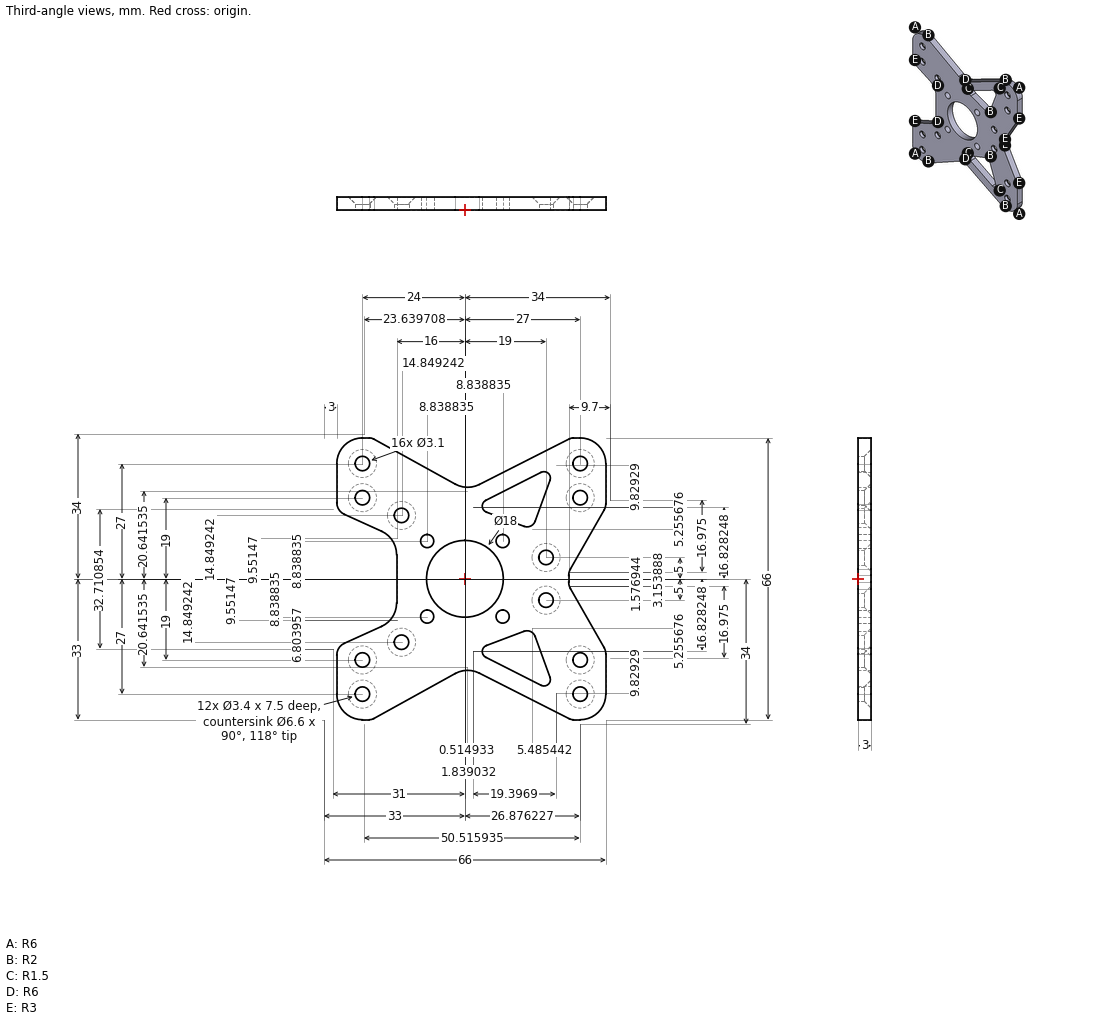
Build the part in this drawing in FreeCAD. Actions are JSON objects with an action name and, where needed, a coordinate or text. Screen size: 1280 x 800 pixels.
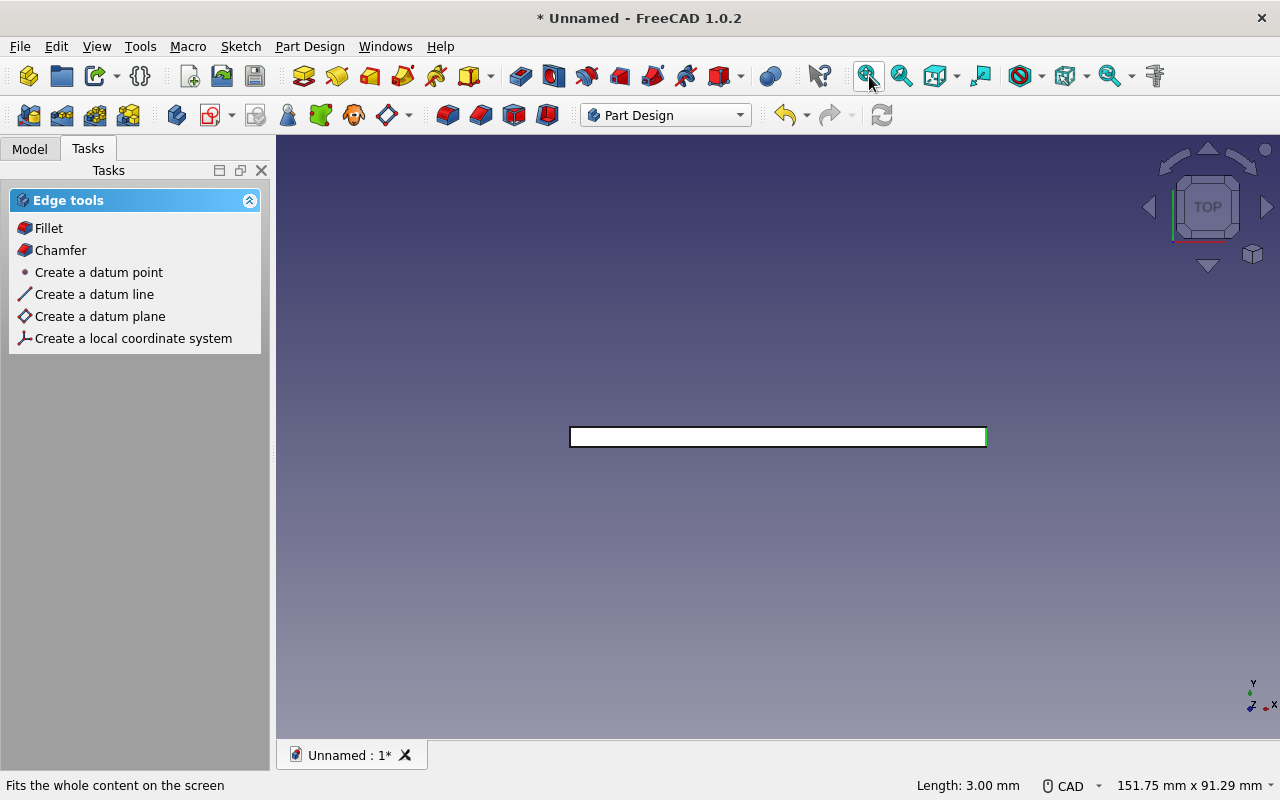
{"action": "key", "text": "v f"}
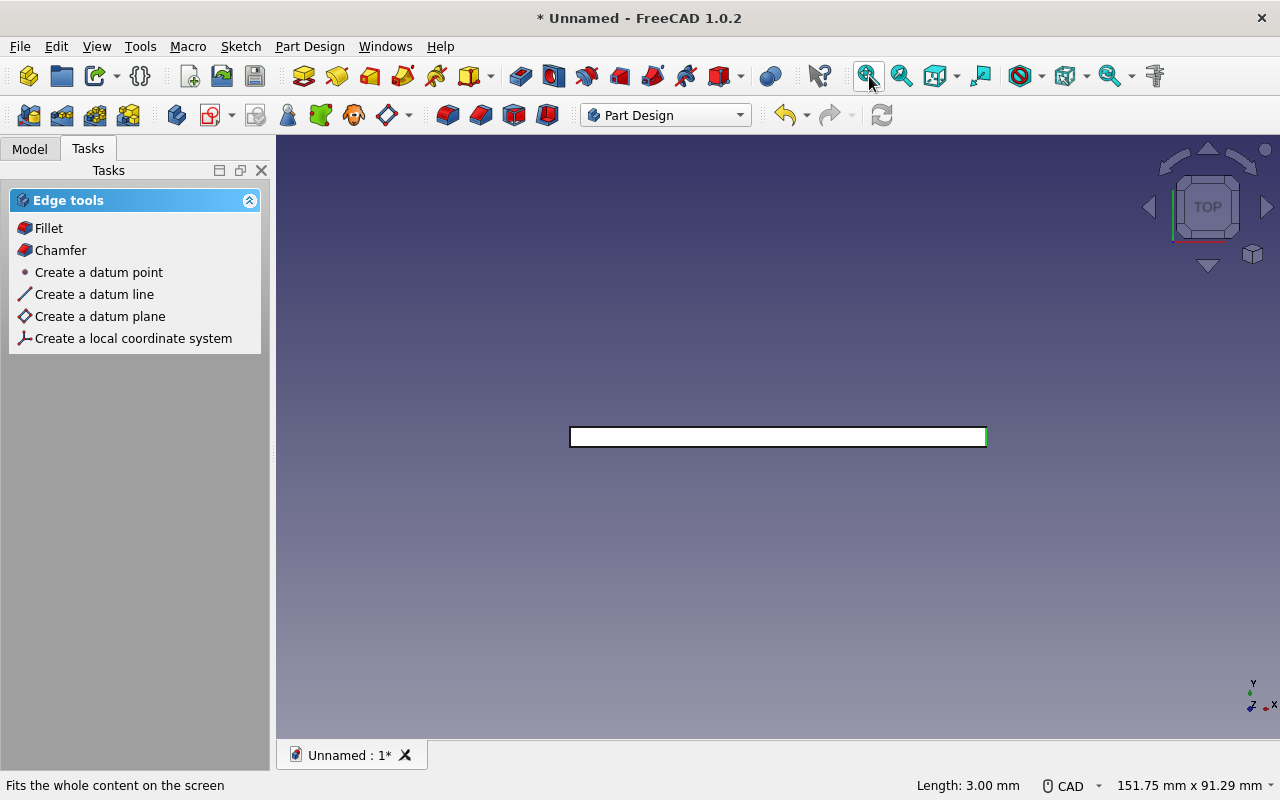
{"action": "left_click", "coordinate": [570, 436], "text": "ctrl"}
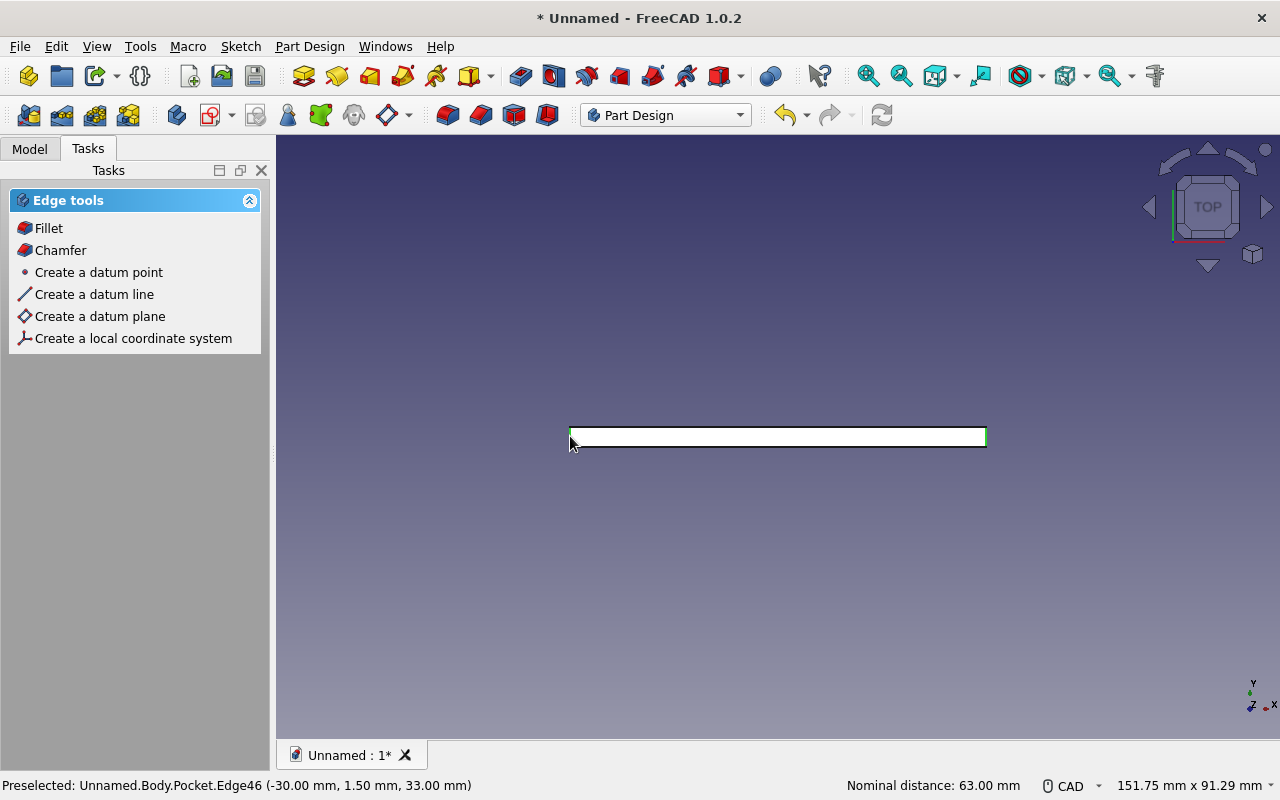
{"action": "scroll", "coordinate": [570, 436], "scroll_direction": "up", "scroll_amount": 4}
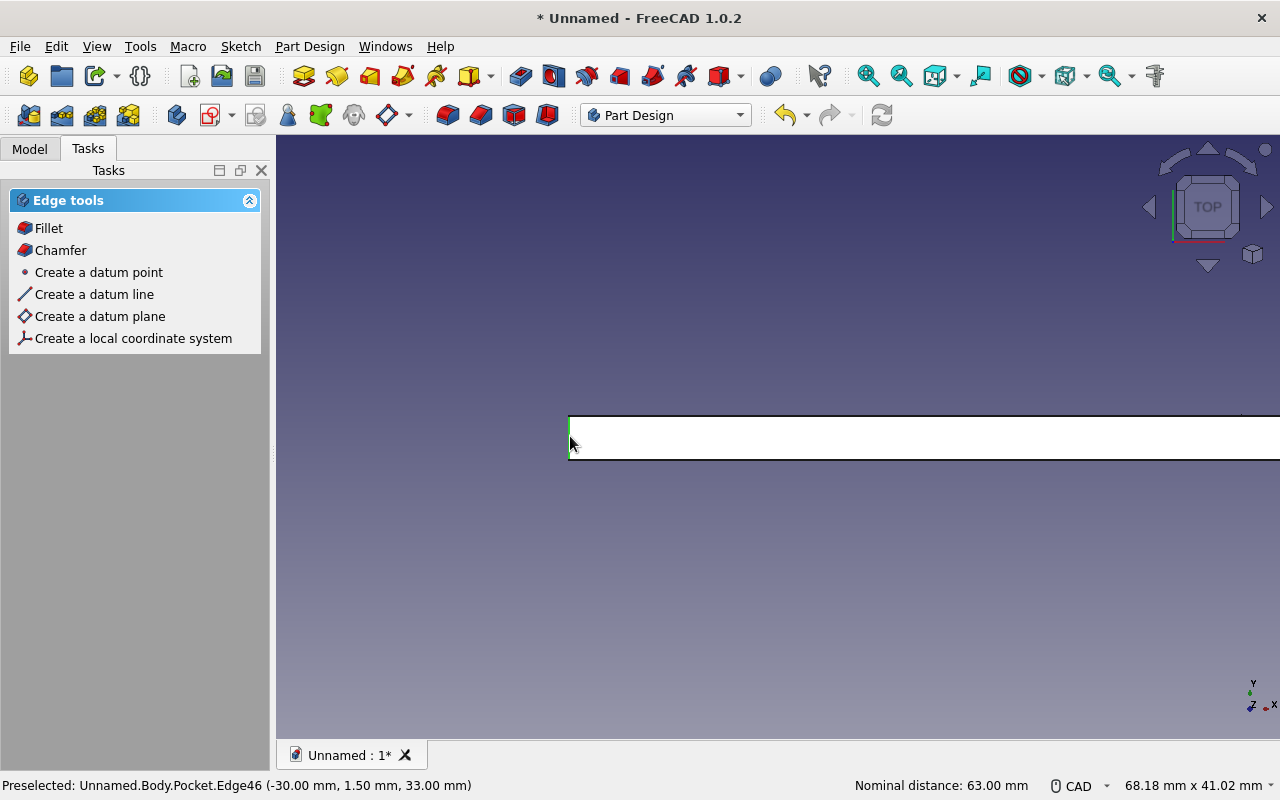
{"action": "left_click", "coordinate": [869, 76]}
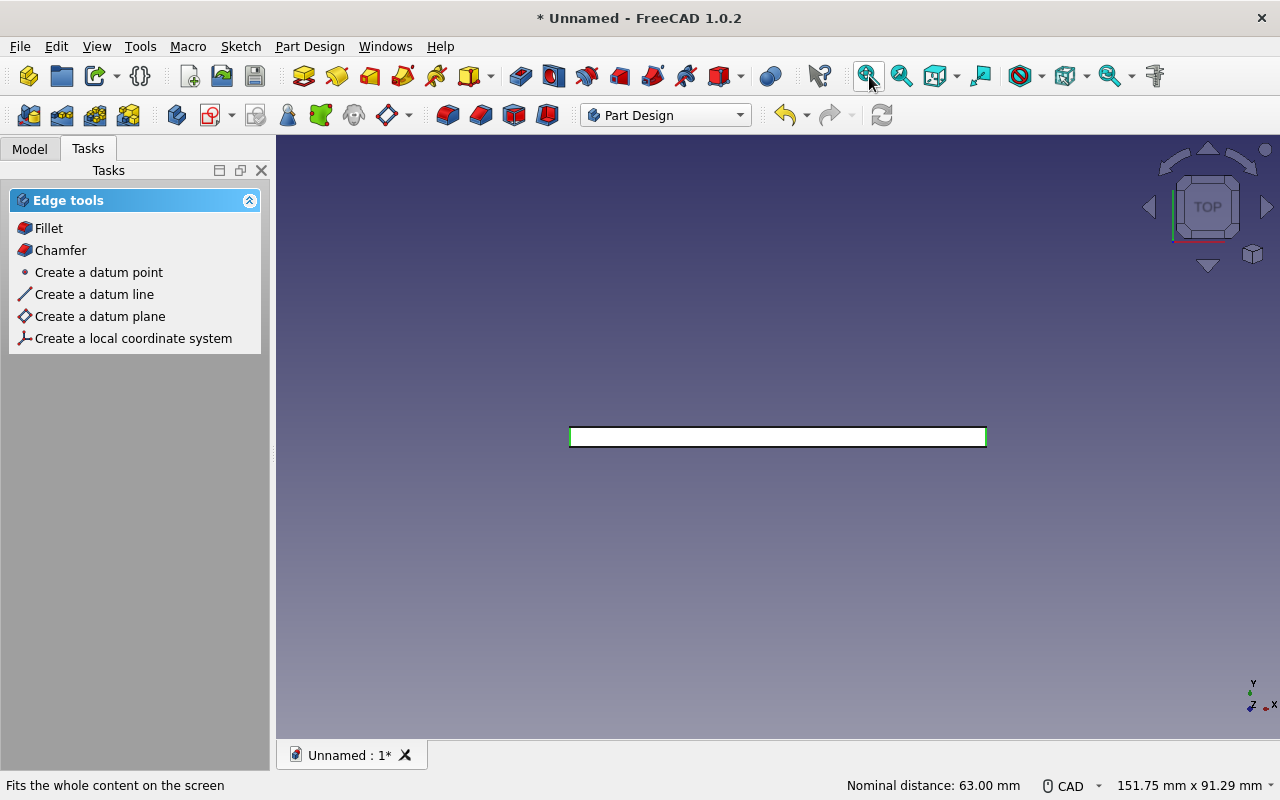
{"action": "key", "text": "1"}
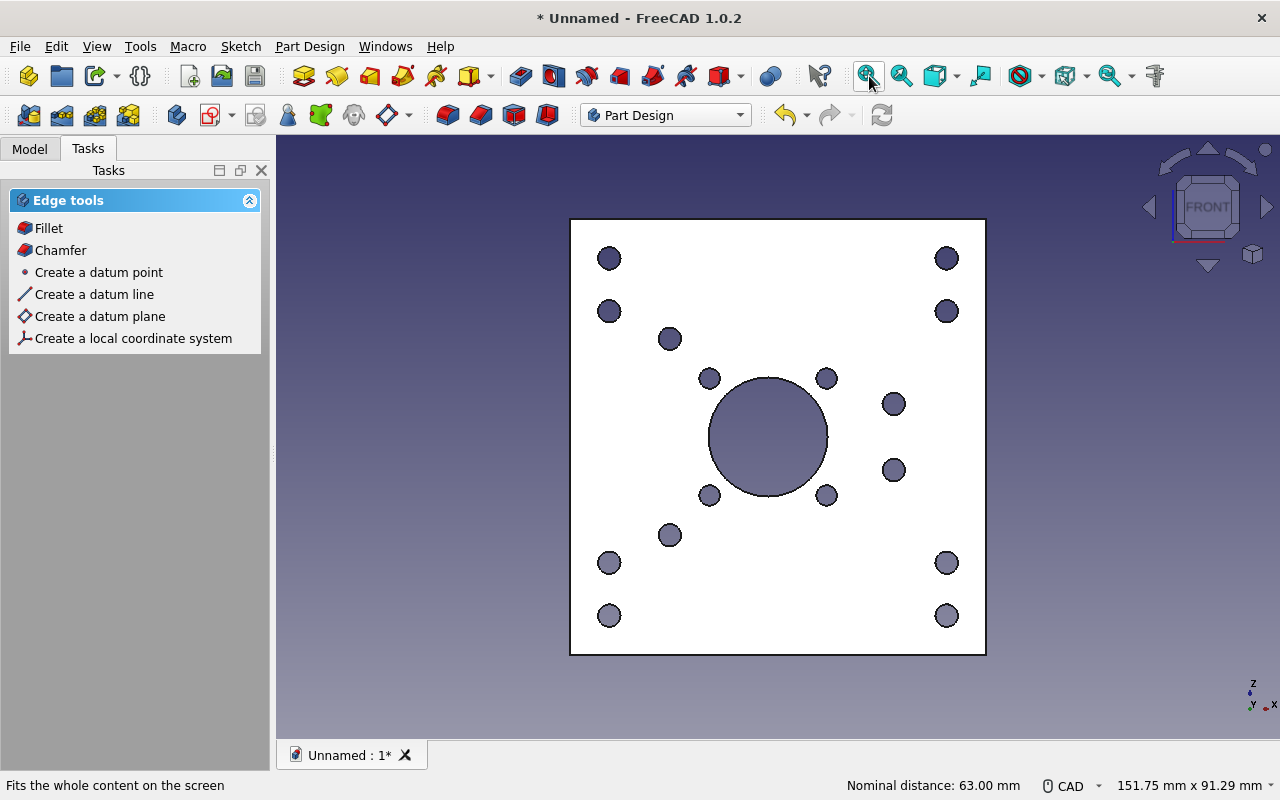
{"action": "scroll", "coordinate": [570, 654], "scroll_direction": "up", "scroll_amount": 4}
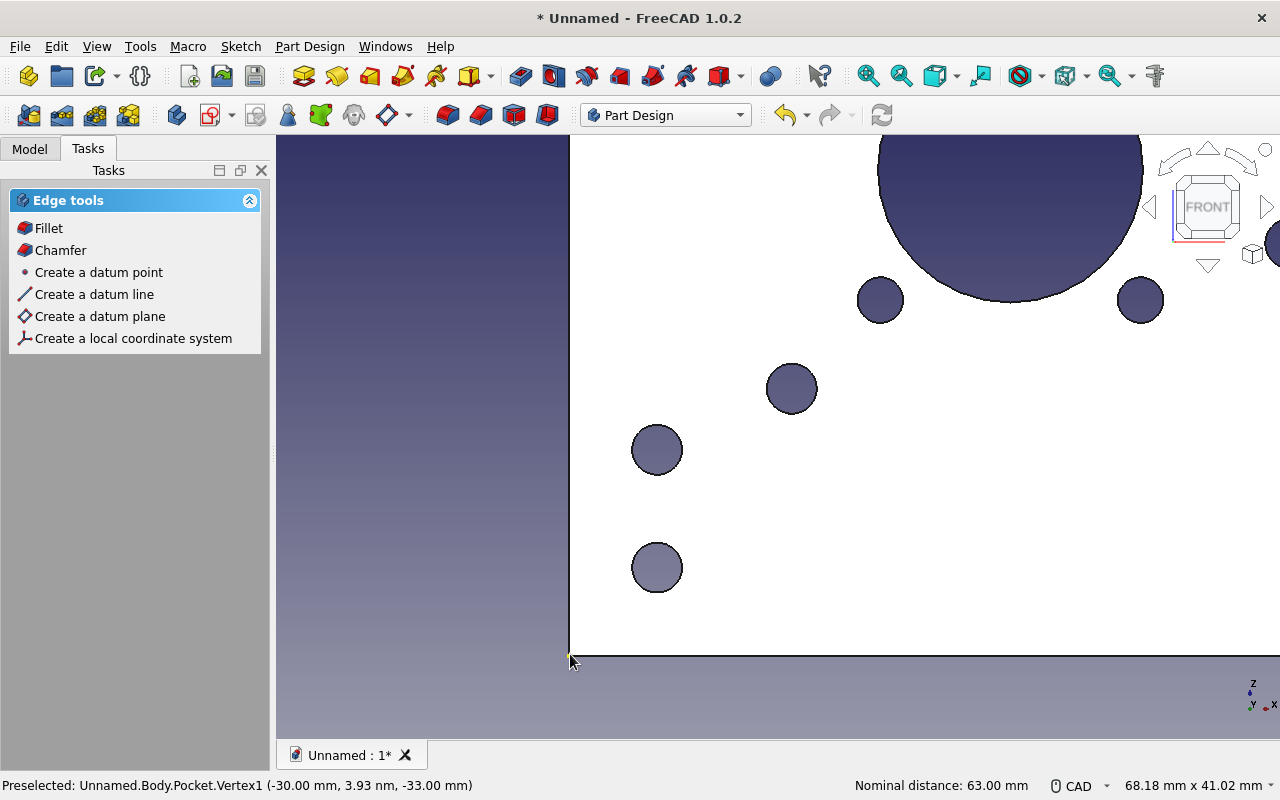
{"action": "left_click", "coordinate": [869, 76]}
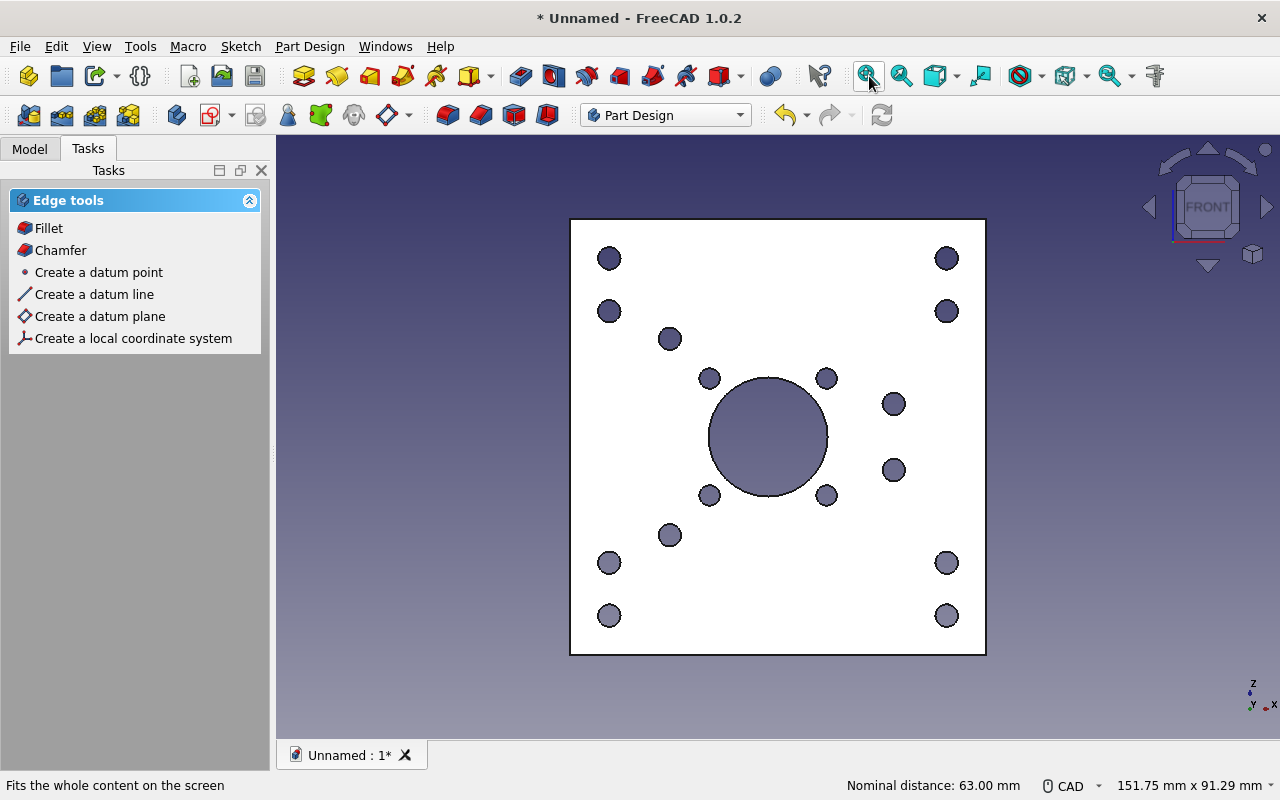
{"action": "key", "text": "3"}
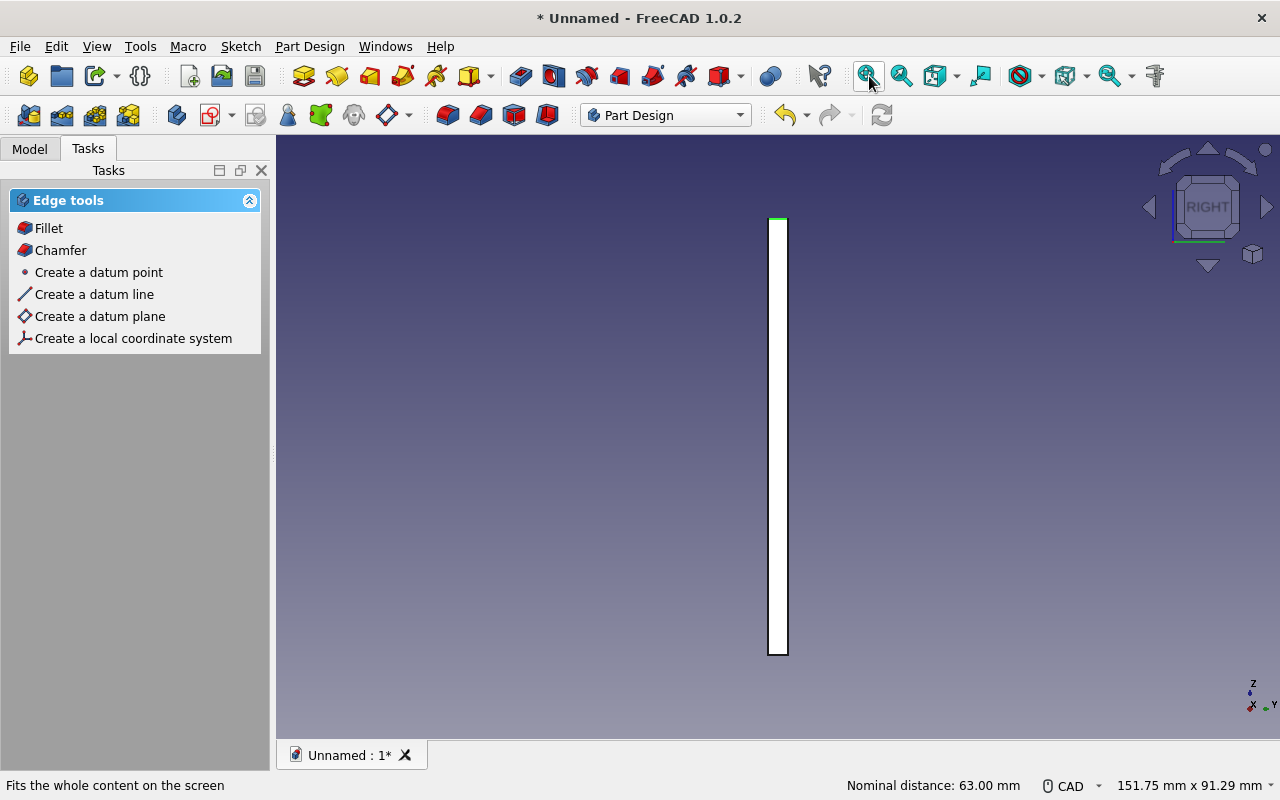
{"action": "left_click", "coordinate": [778, 654], "text": "ctrl"}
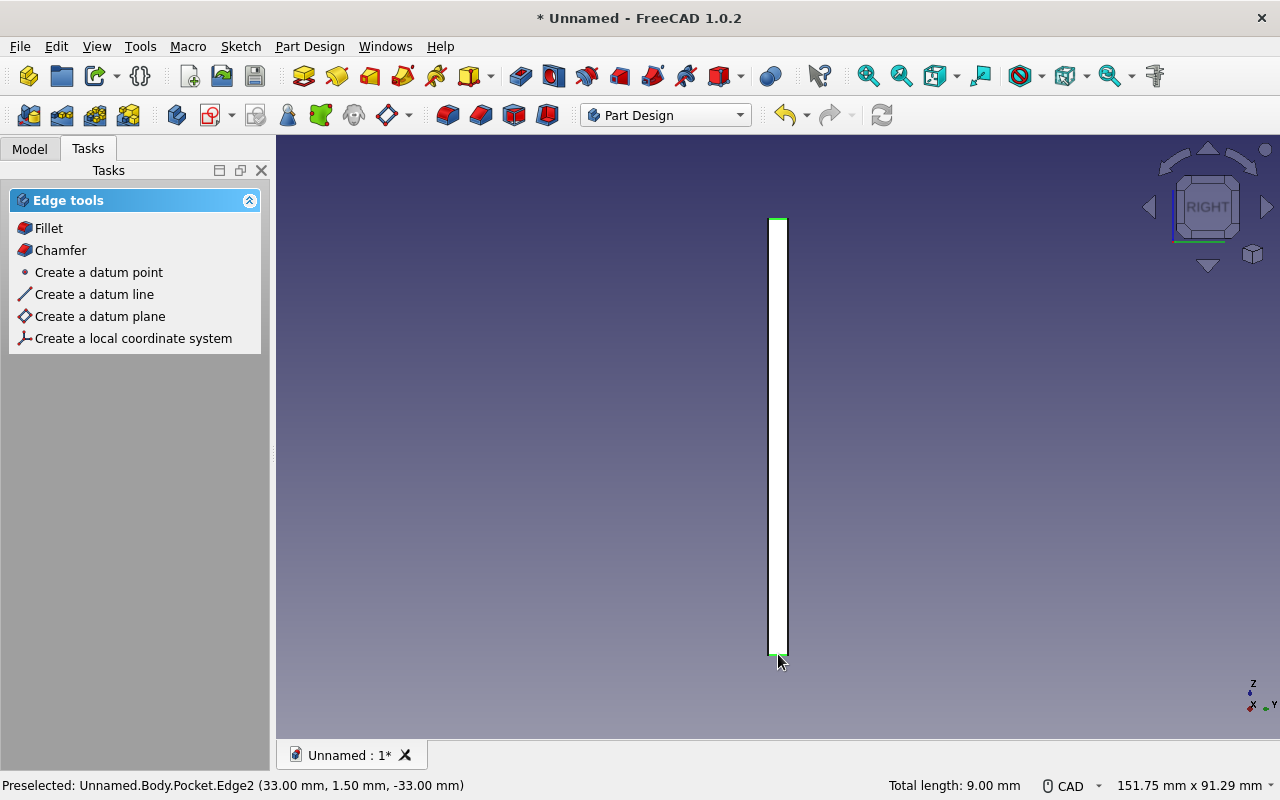
{"action": "scroll", "coordinate": [778, 654], "scroll_direction": "up", "scroll_amount": 4}